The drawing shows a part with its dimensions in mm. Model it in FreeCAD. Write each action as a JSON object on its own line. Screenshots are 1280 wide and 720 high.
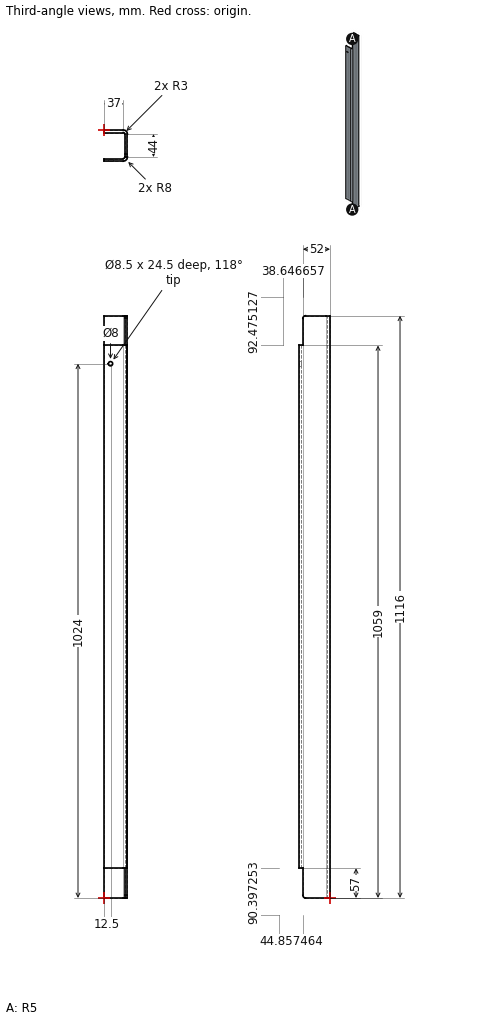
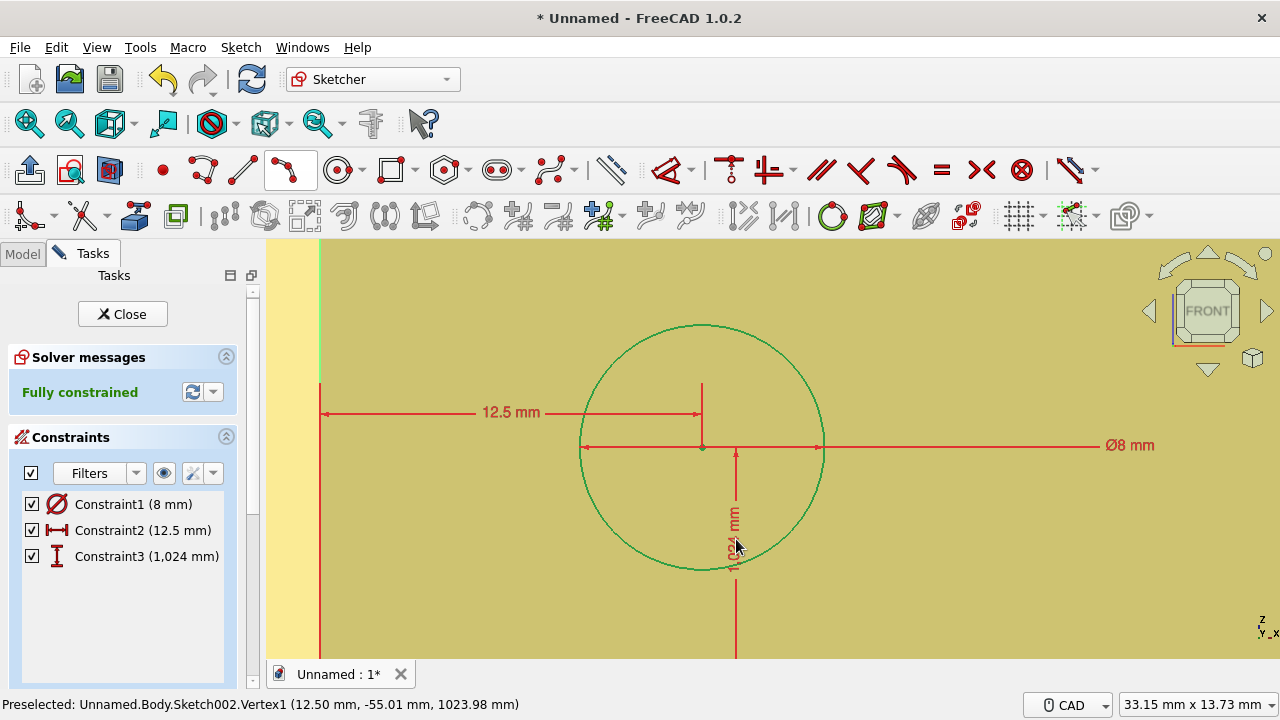
{"action": "left_click", "coordinate": [123, 314]}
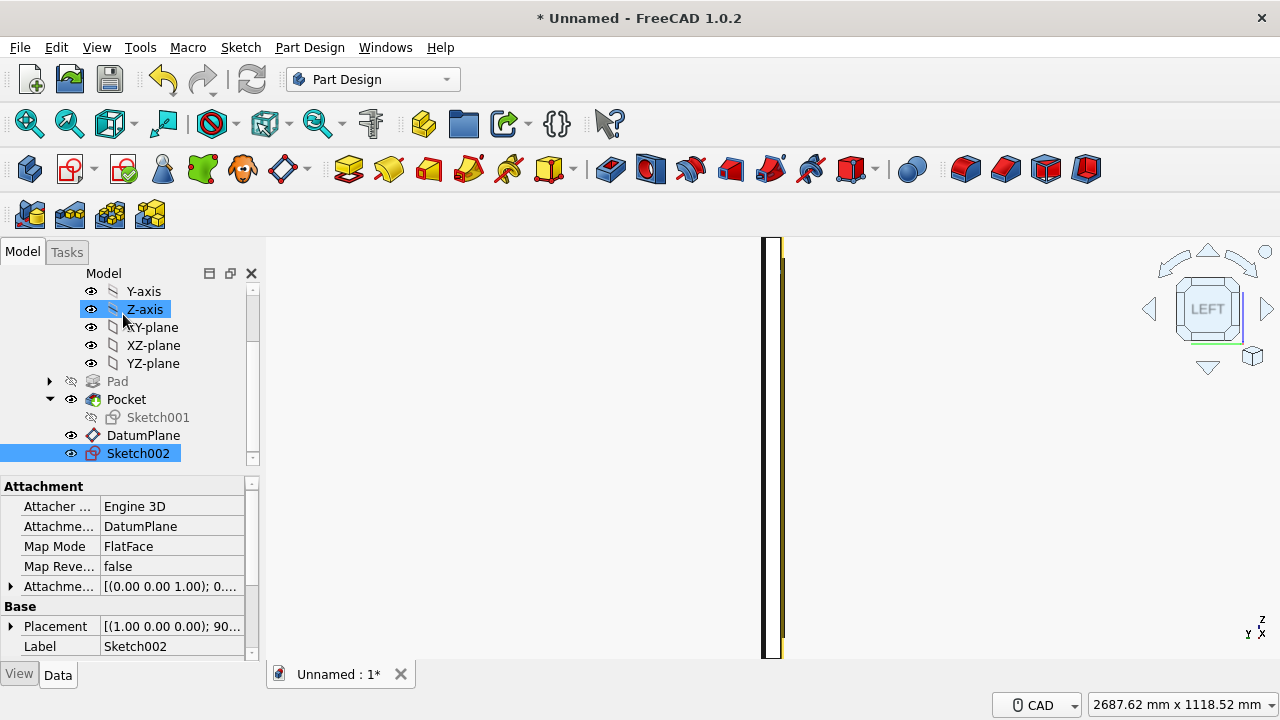
{"action": "left_click", "coordinate": [612, 170]}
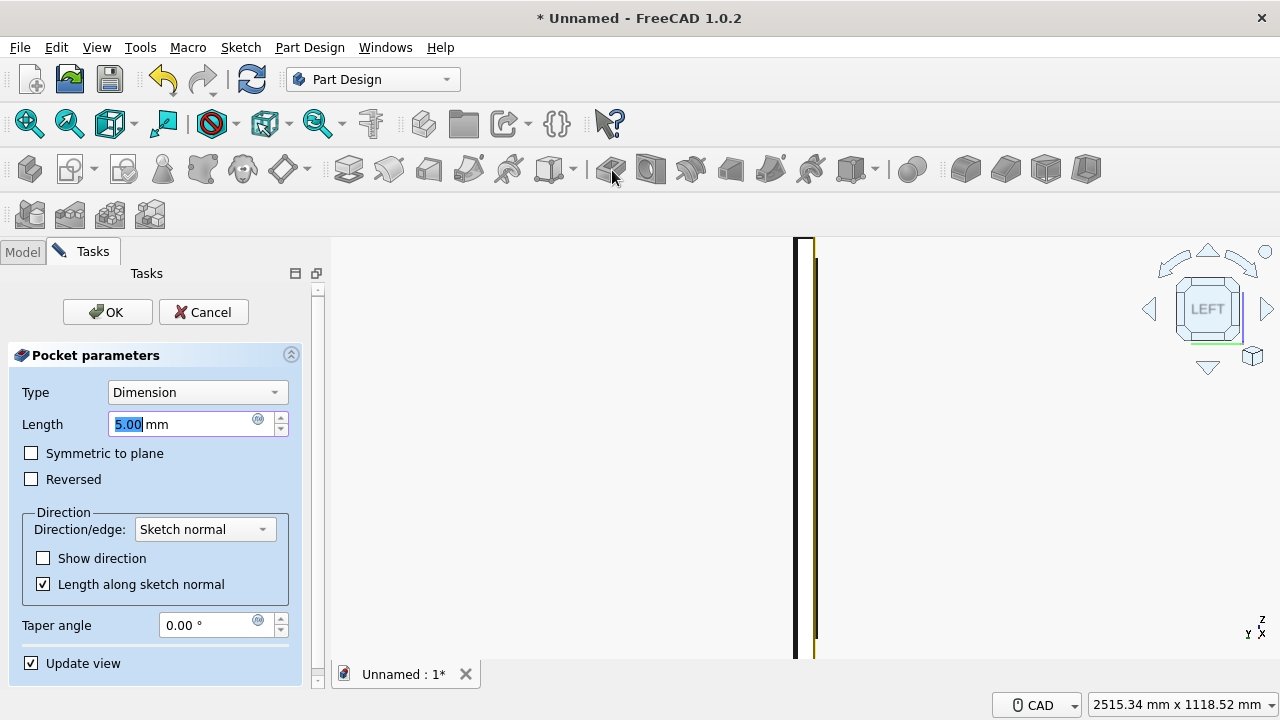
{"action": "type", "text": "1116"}
{"action": "key", "text": "Tab"}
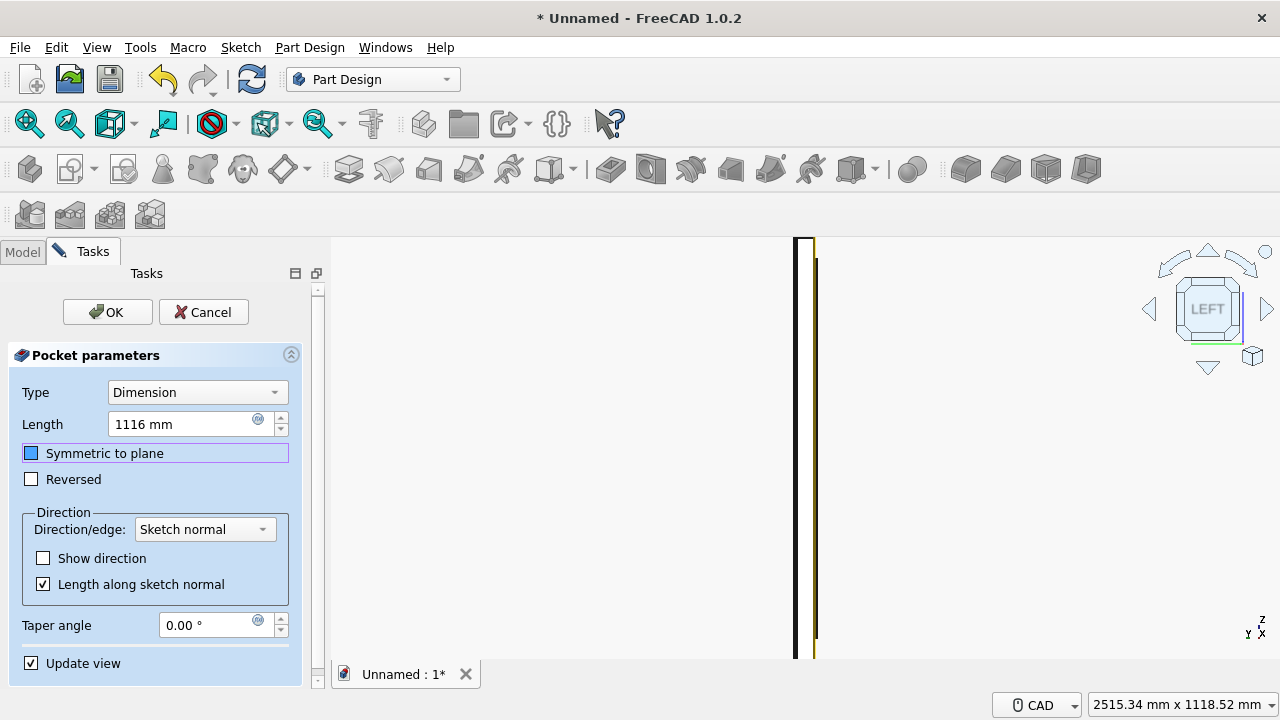
{"action": "left_click", "coordinate": [30, 479]}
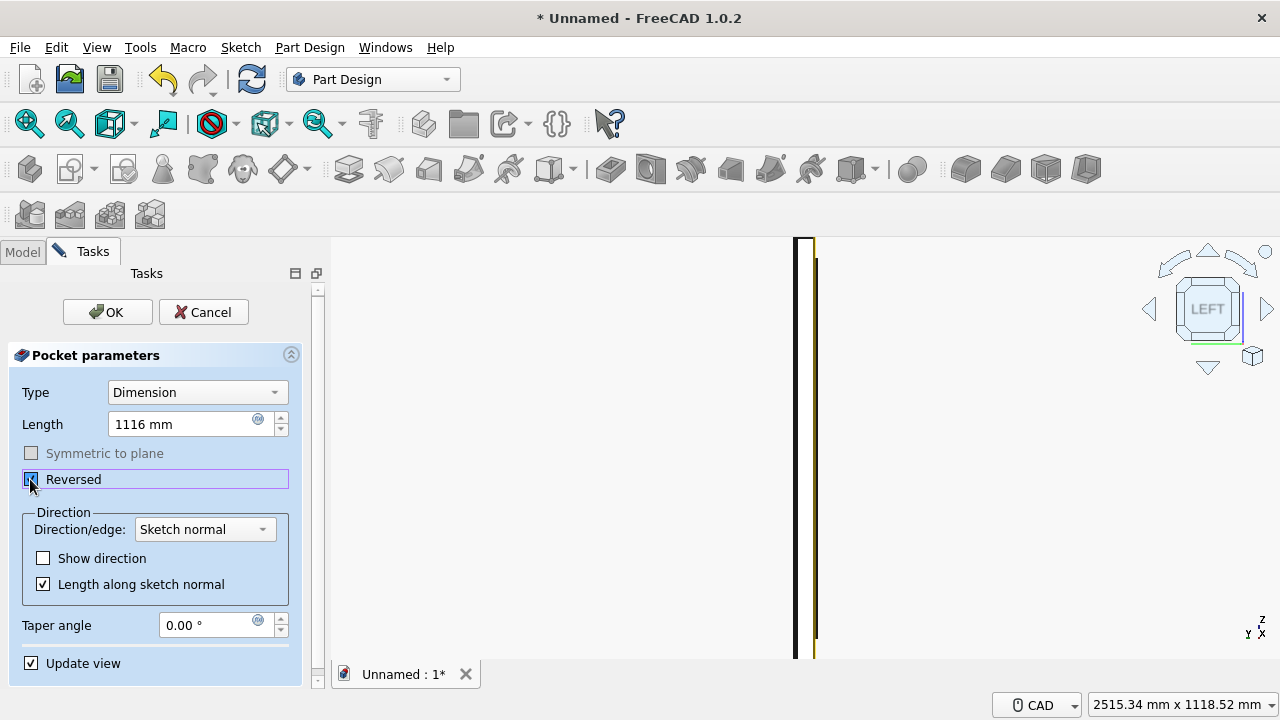
{"action": "left_click", "coordinate": [108, 312]}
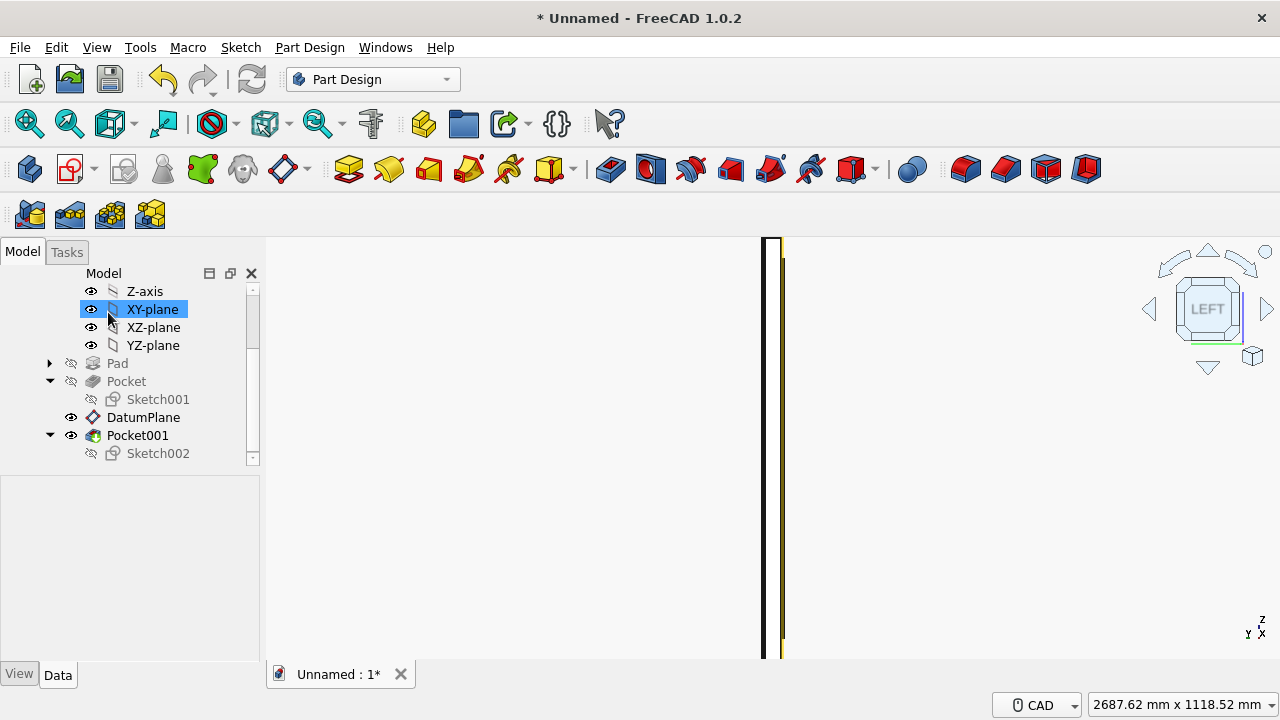
{"action": "left_click", "coordinate": [116, 417]}
{"action": "key", "text": "space"}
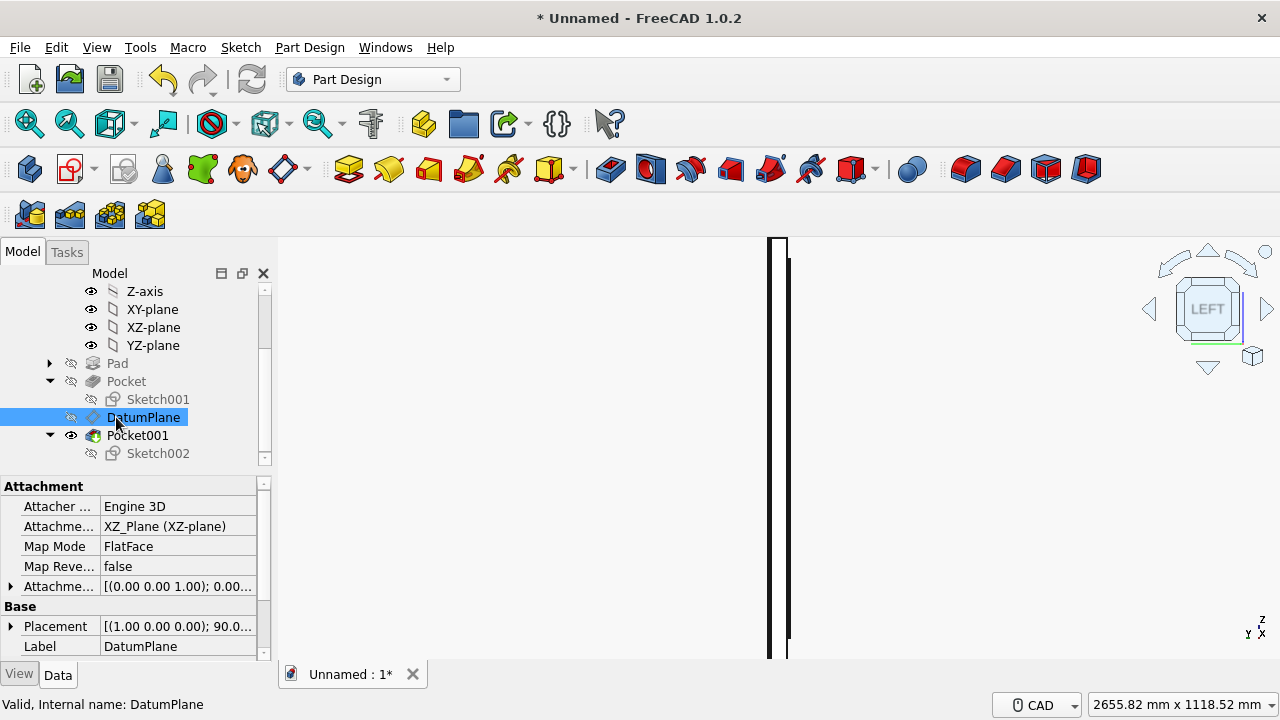
{"action": "key", "text": "0"}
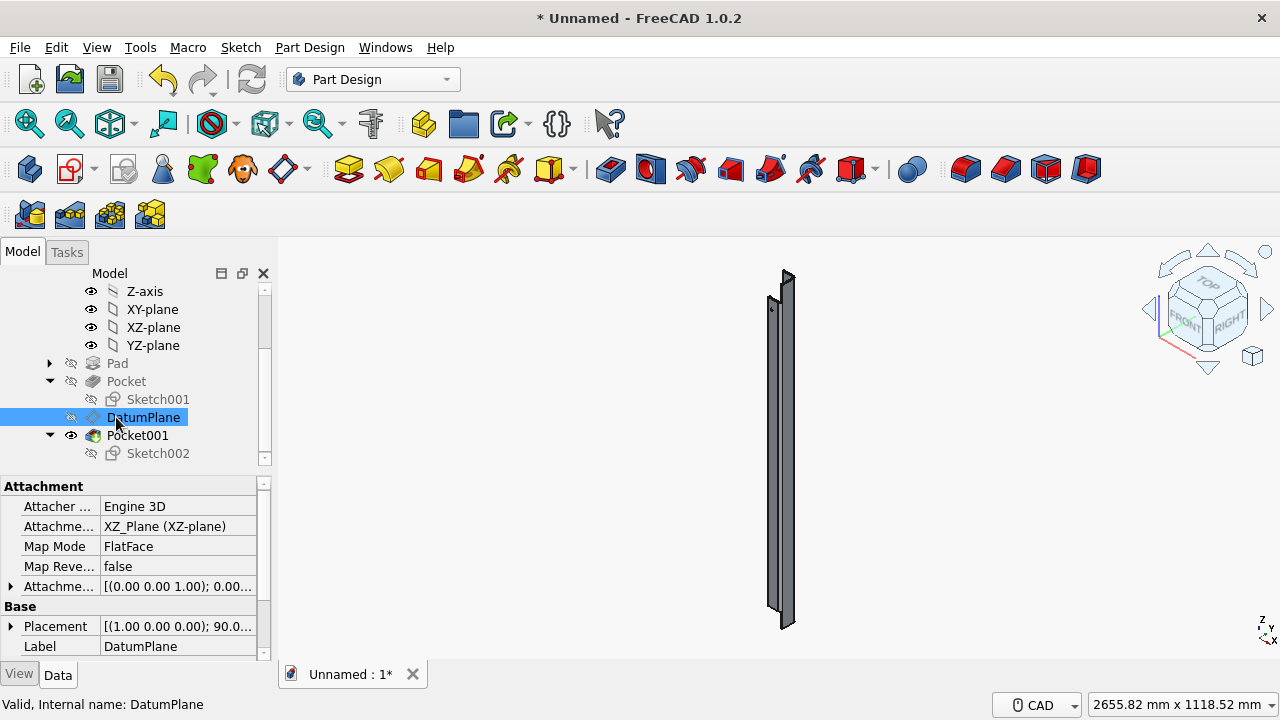
{"action": "scroll", "coordinate": [782, 628], "scroll_direction": "up", "scroll_amount": 15}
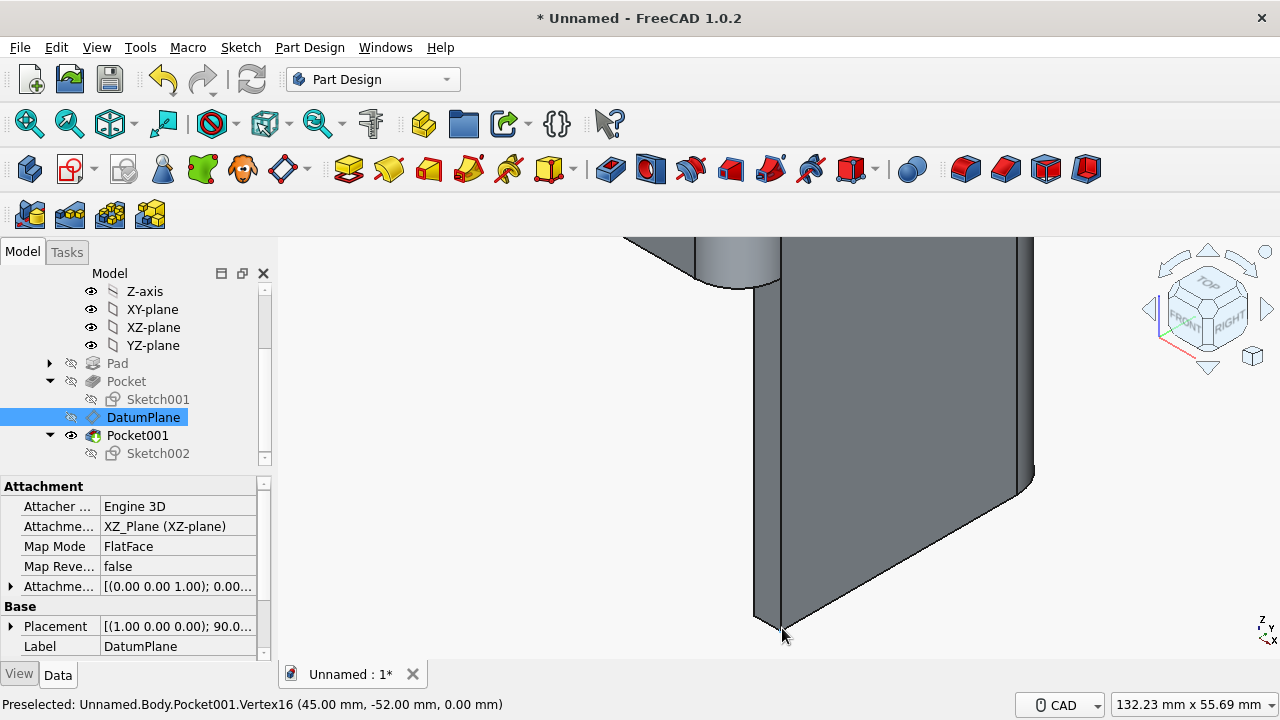
{"action": "key", "text": "v f"}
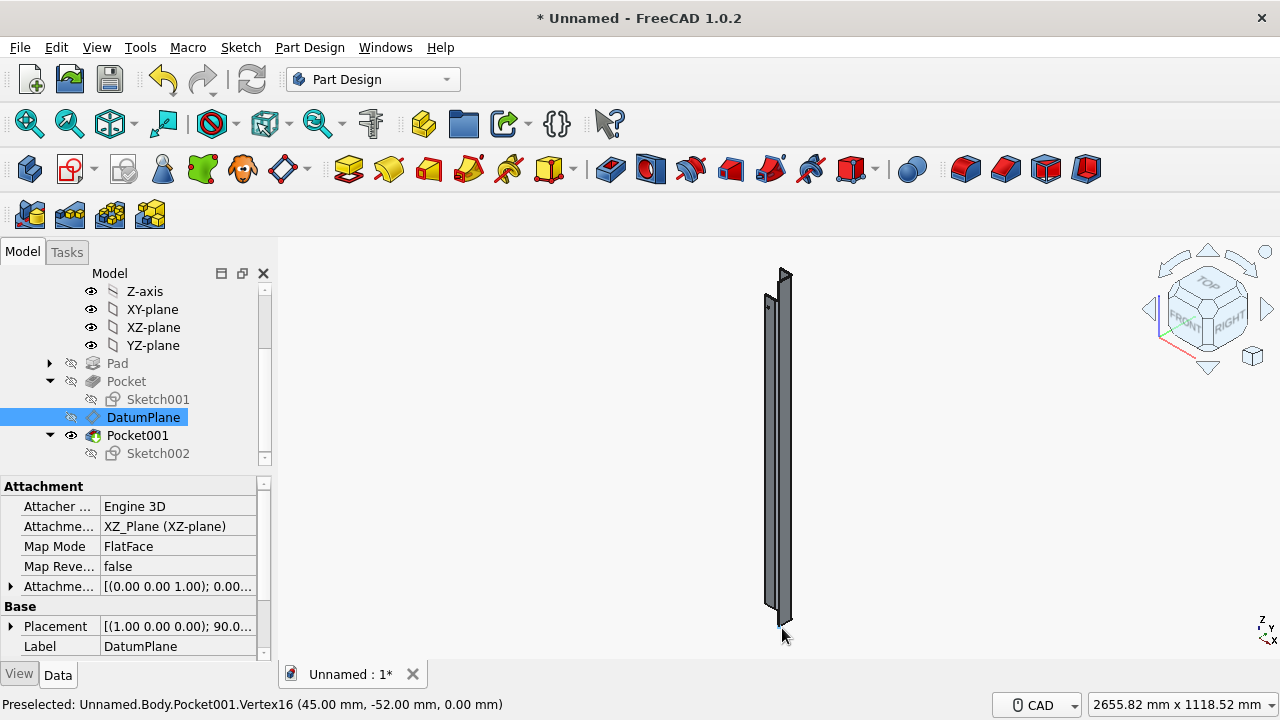
{"action": "key", "text": "2"}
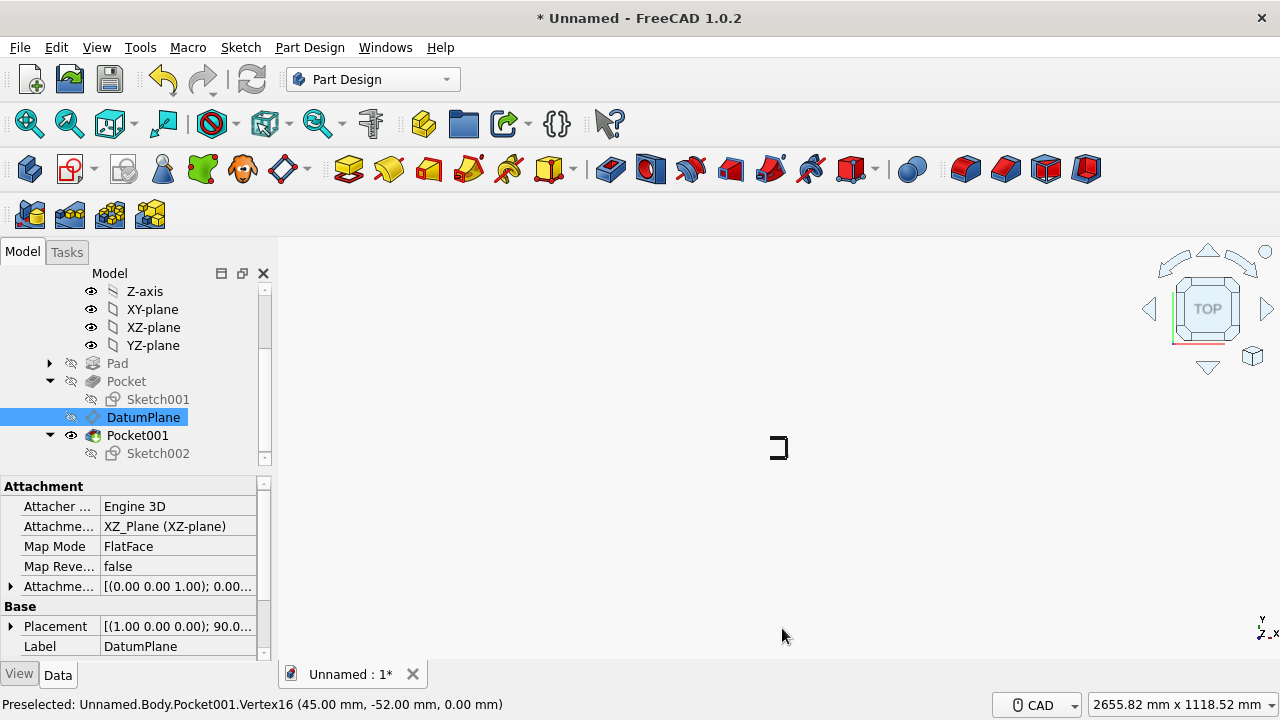
{"action": "left_click", "coordinate": [30, 124]}